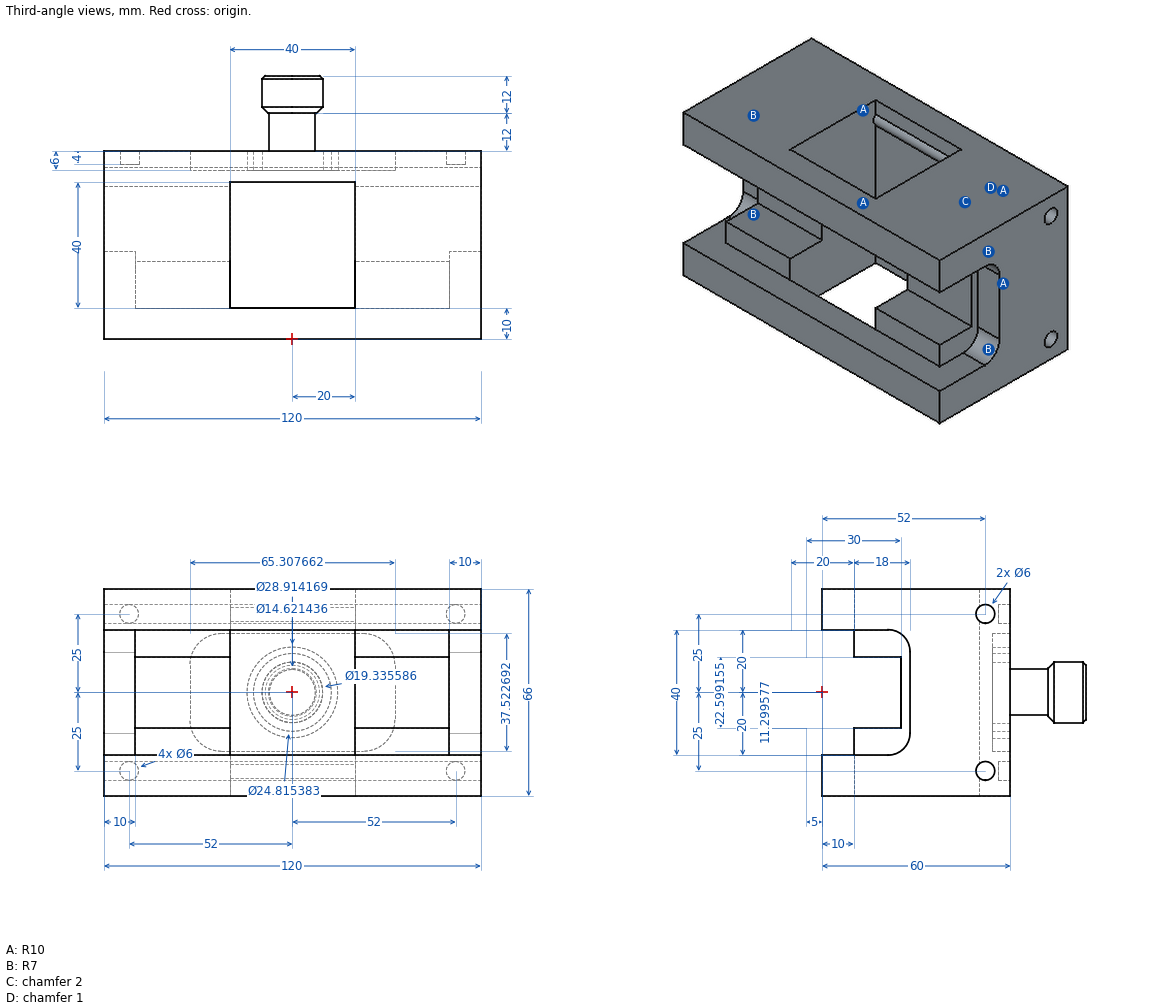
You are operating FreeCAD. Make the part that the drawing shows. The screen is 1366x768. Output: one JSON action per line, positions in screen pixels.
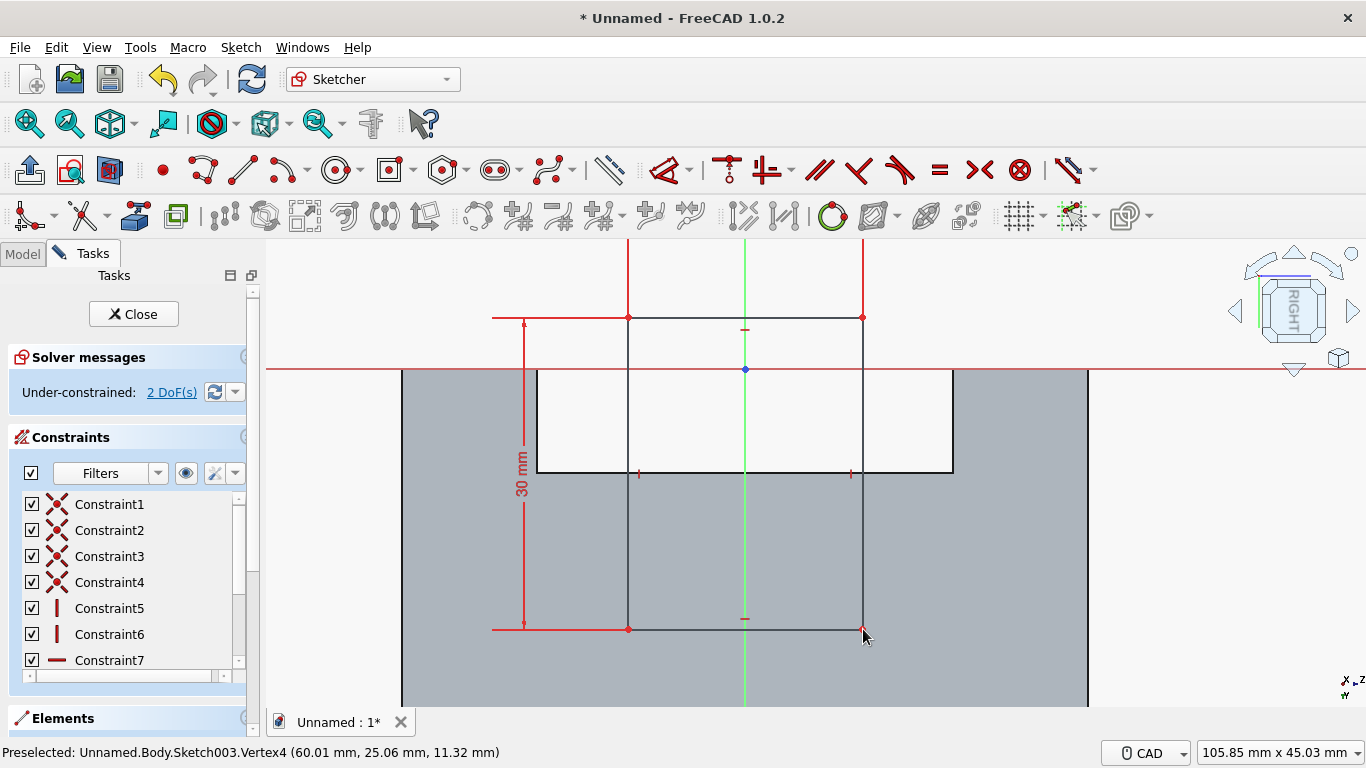
{"action": "left_click", "coordinate": [664, 170]}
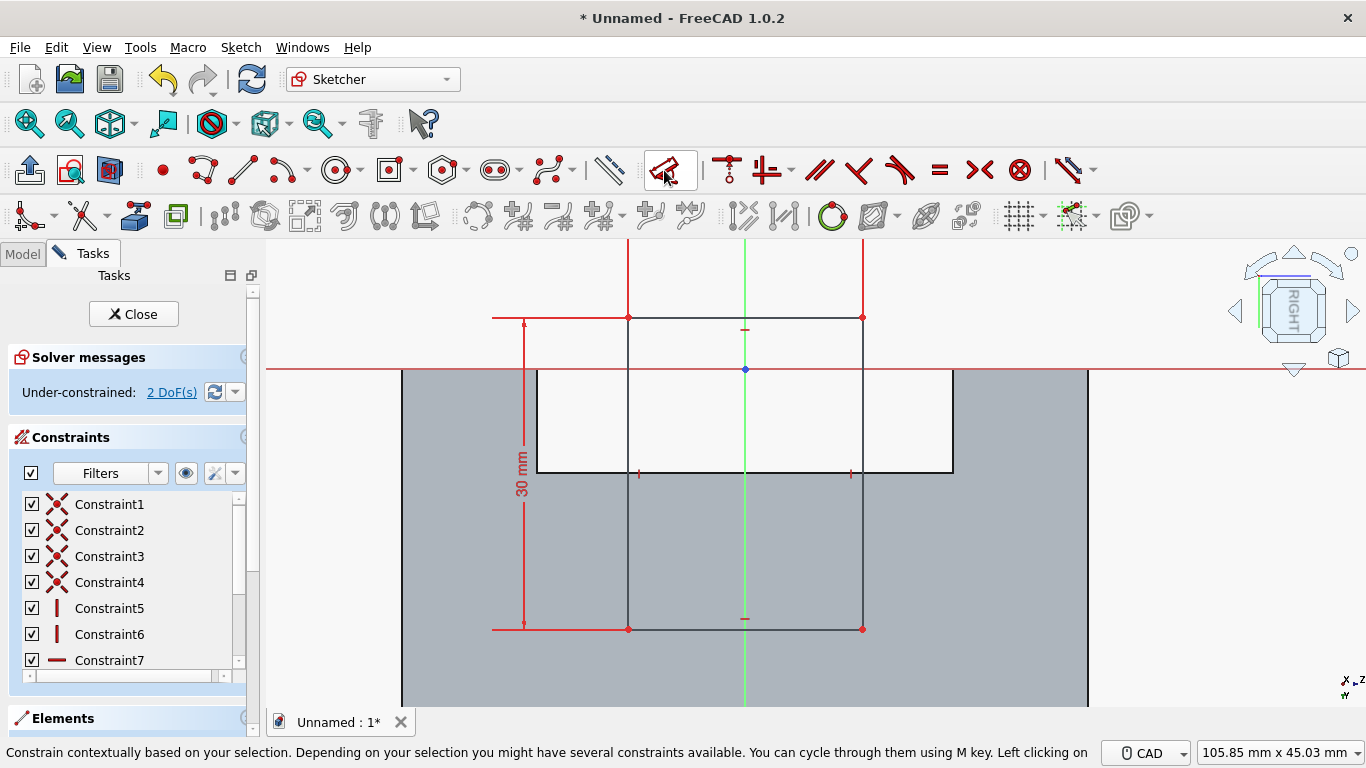
{"action": "left_click", "coordinate": [628, 318]}
{"action": "left_click", "coordinate": [594, 344]}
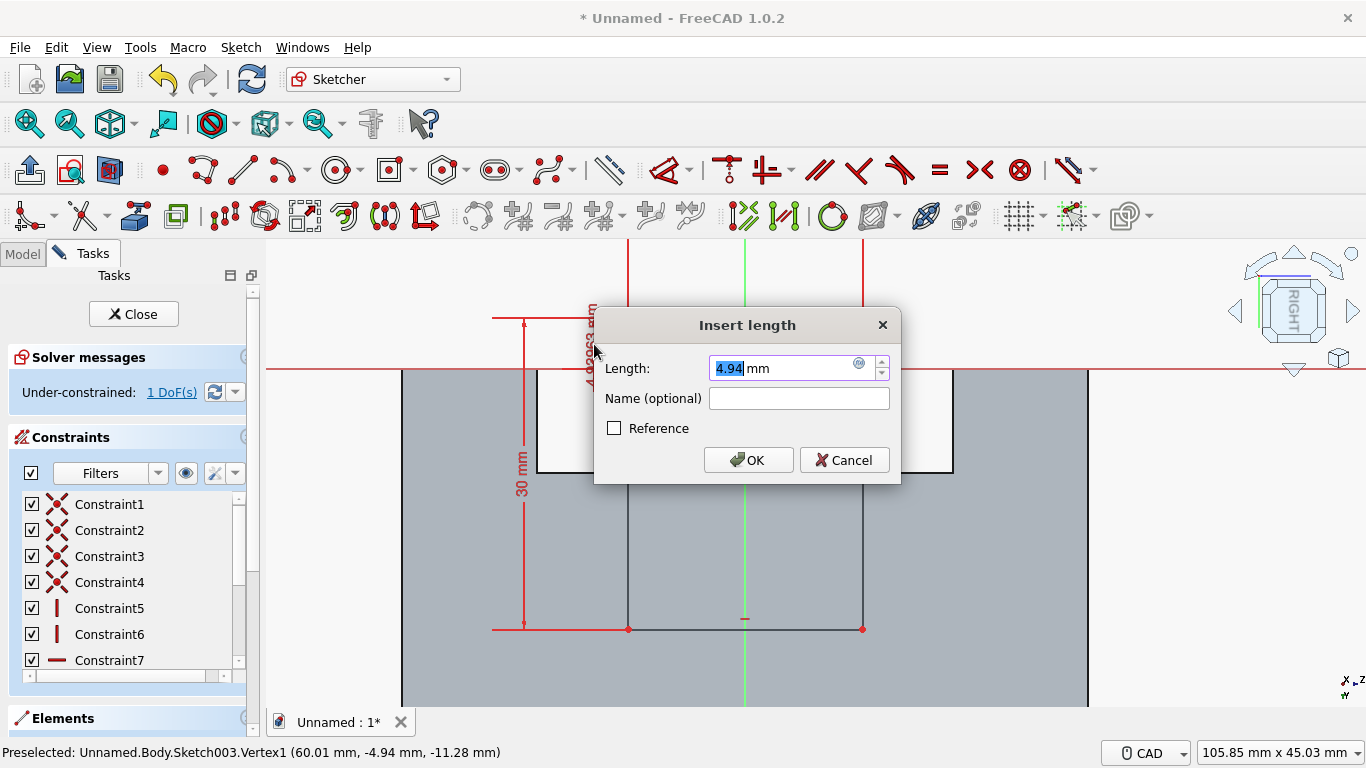
{"action": "type", "text": "5"}
{"action": "key", "text": "Return"}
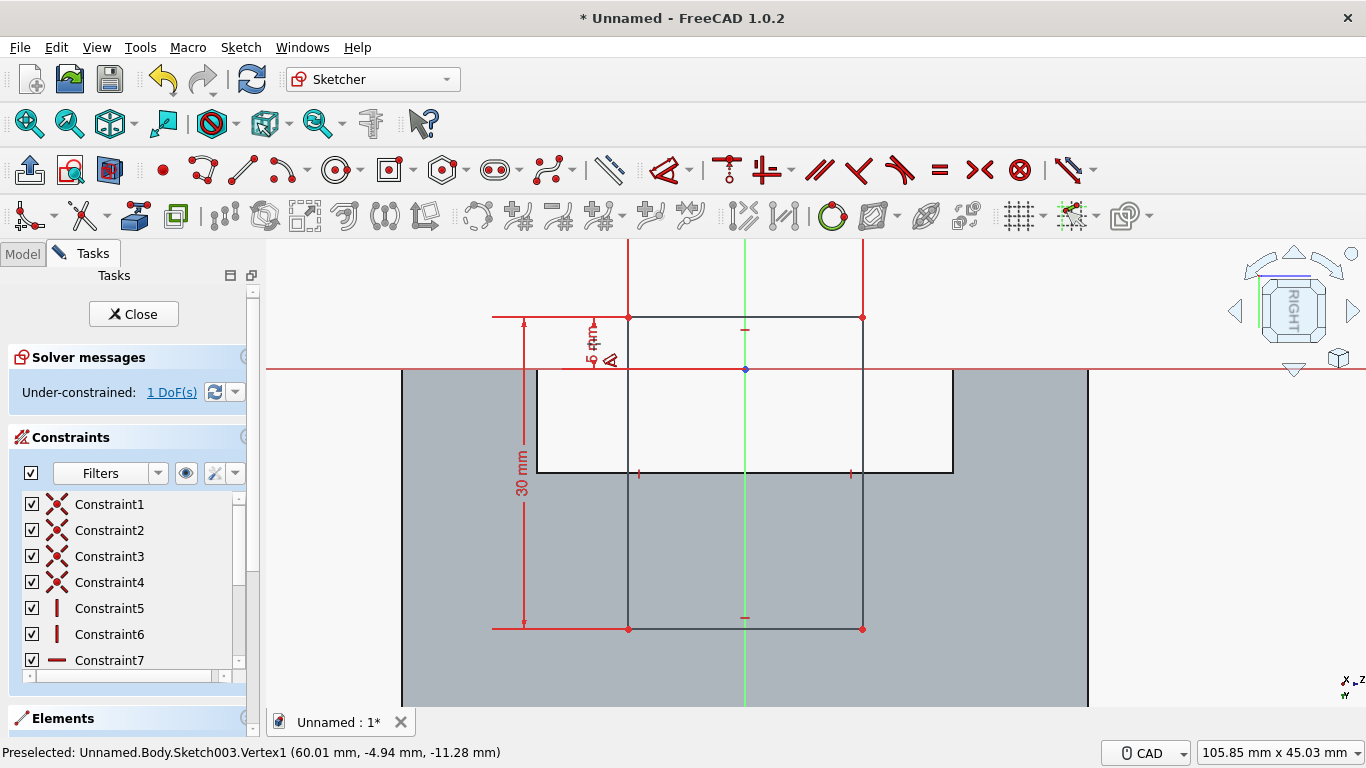
{"action": "left_click", "coordinate": [628, 317]}
{"action": "left_click", "coordinate": [687, 283]}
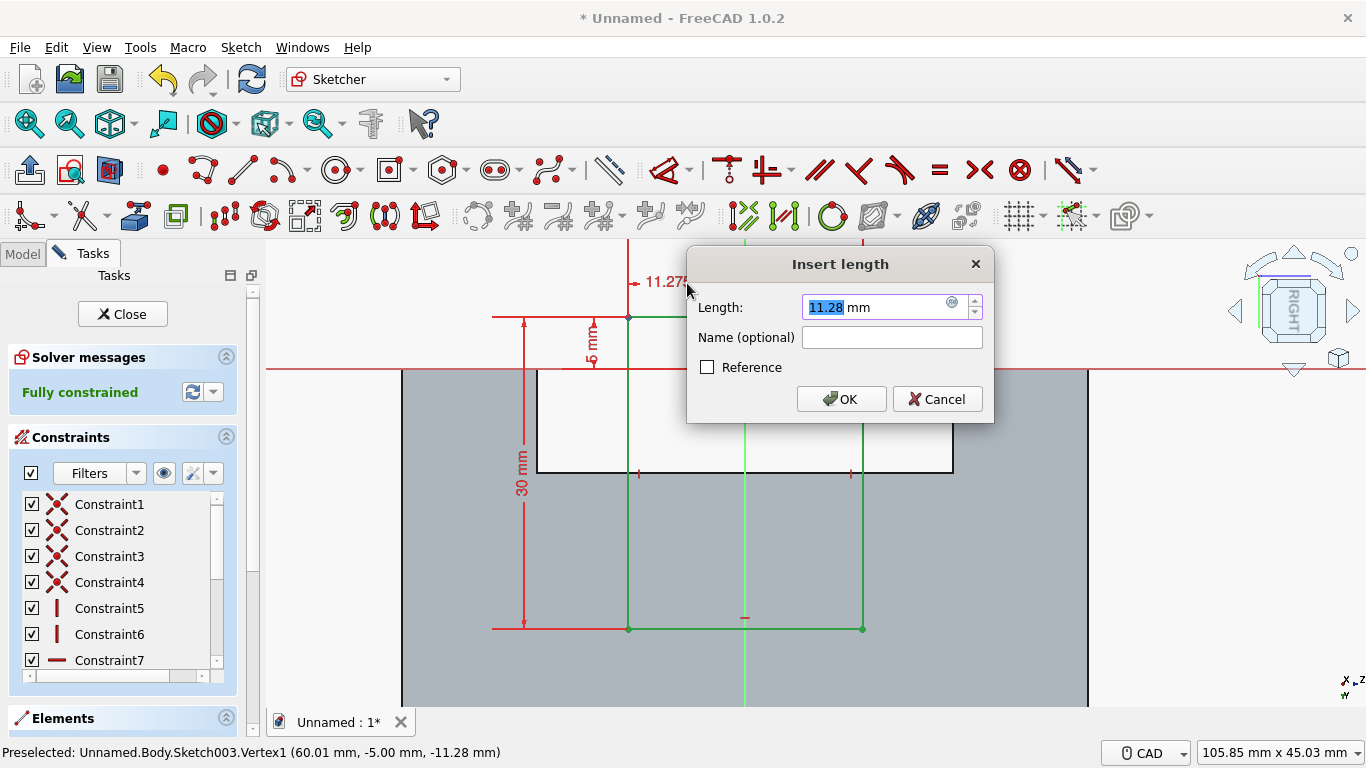
{"action": "type", "text": "11.299577"}
{"action": "key", "text": "Return"}
{"action": "key", "text": "Escape"}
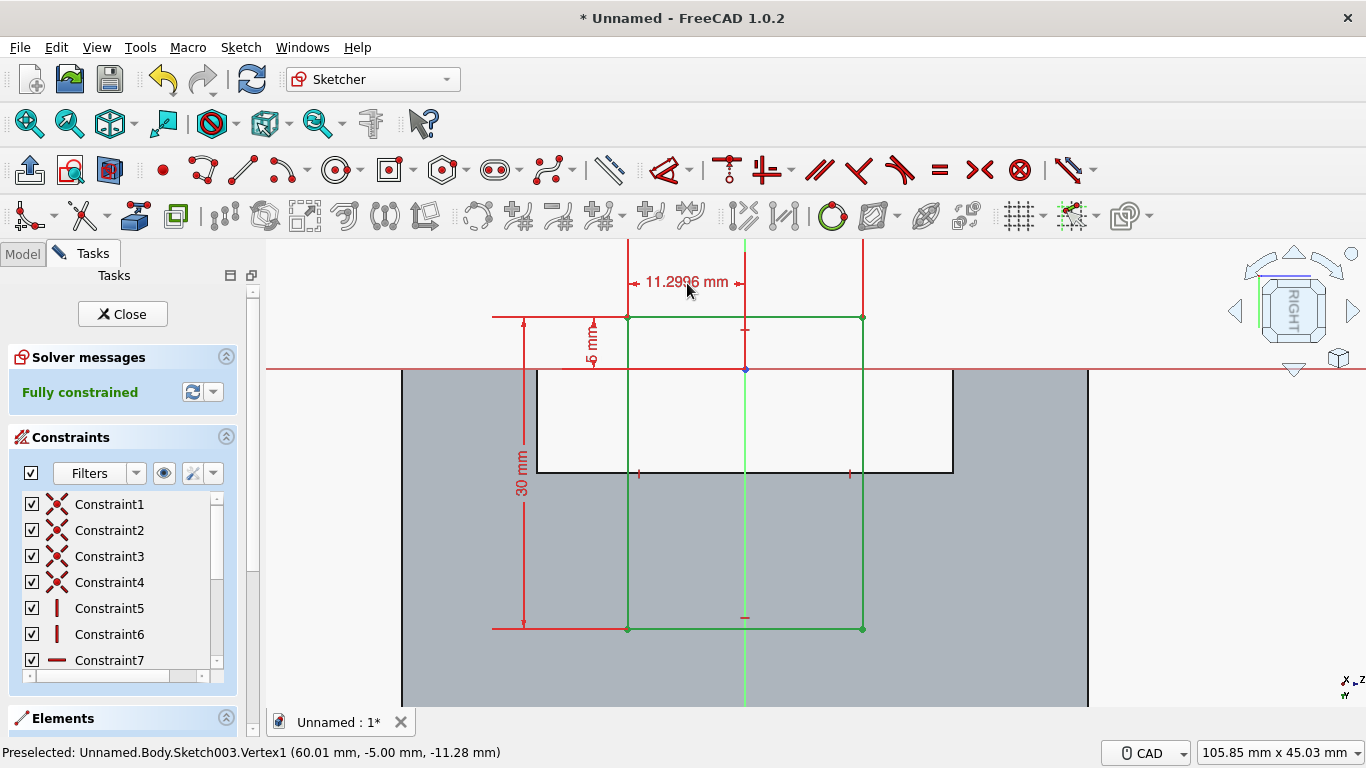
{"action": "left_click", "coordinate": [123, 314]}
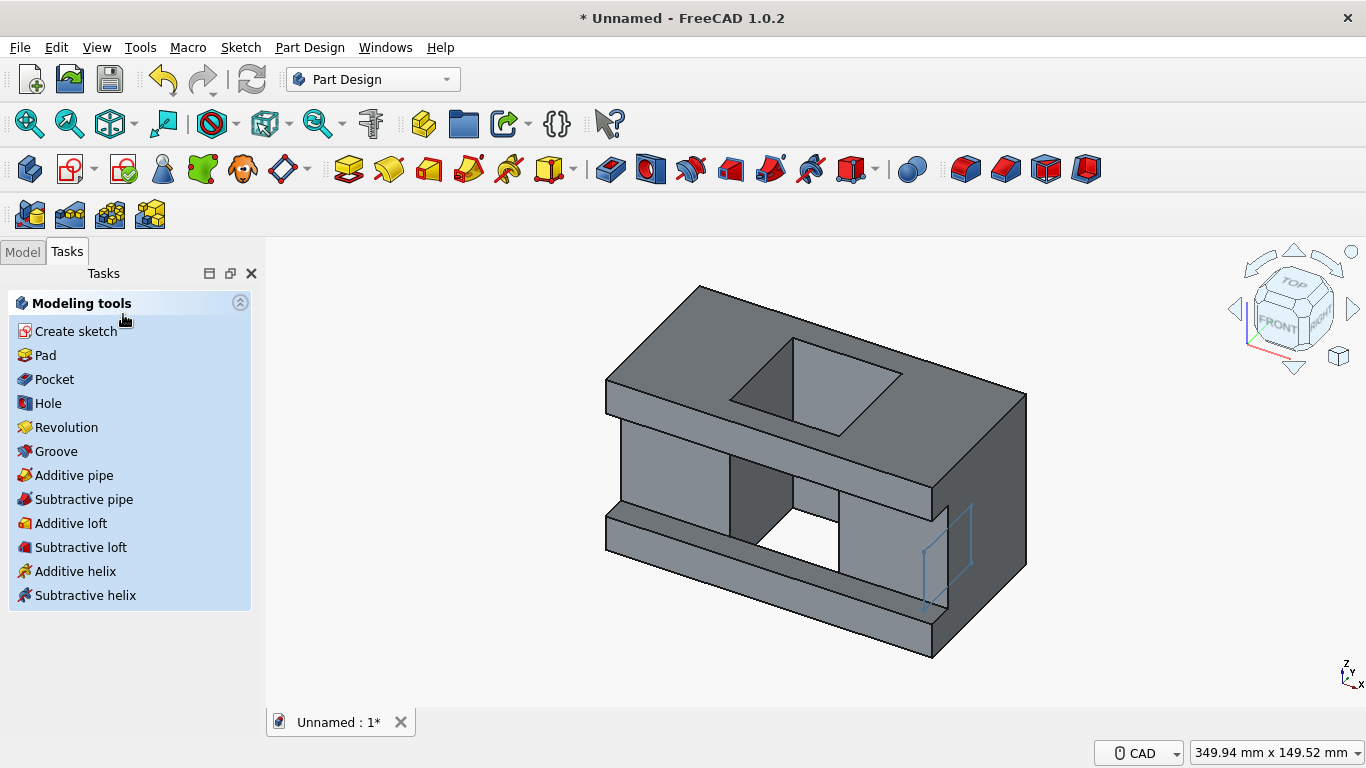
{"action": "left_click", "coordinate": [612, 170]}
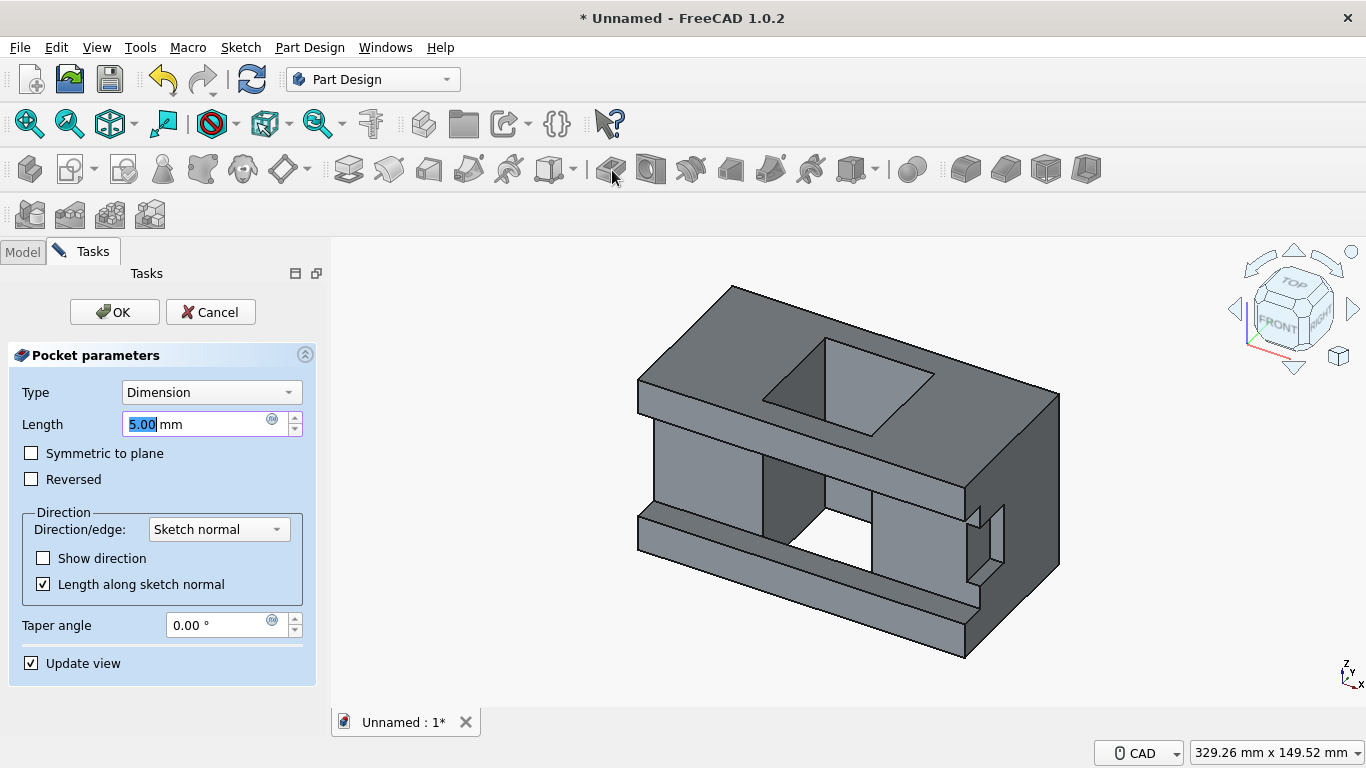
{"action": "type", "text": "120"}
{"action": "key", "text": "Tab"}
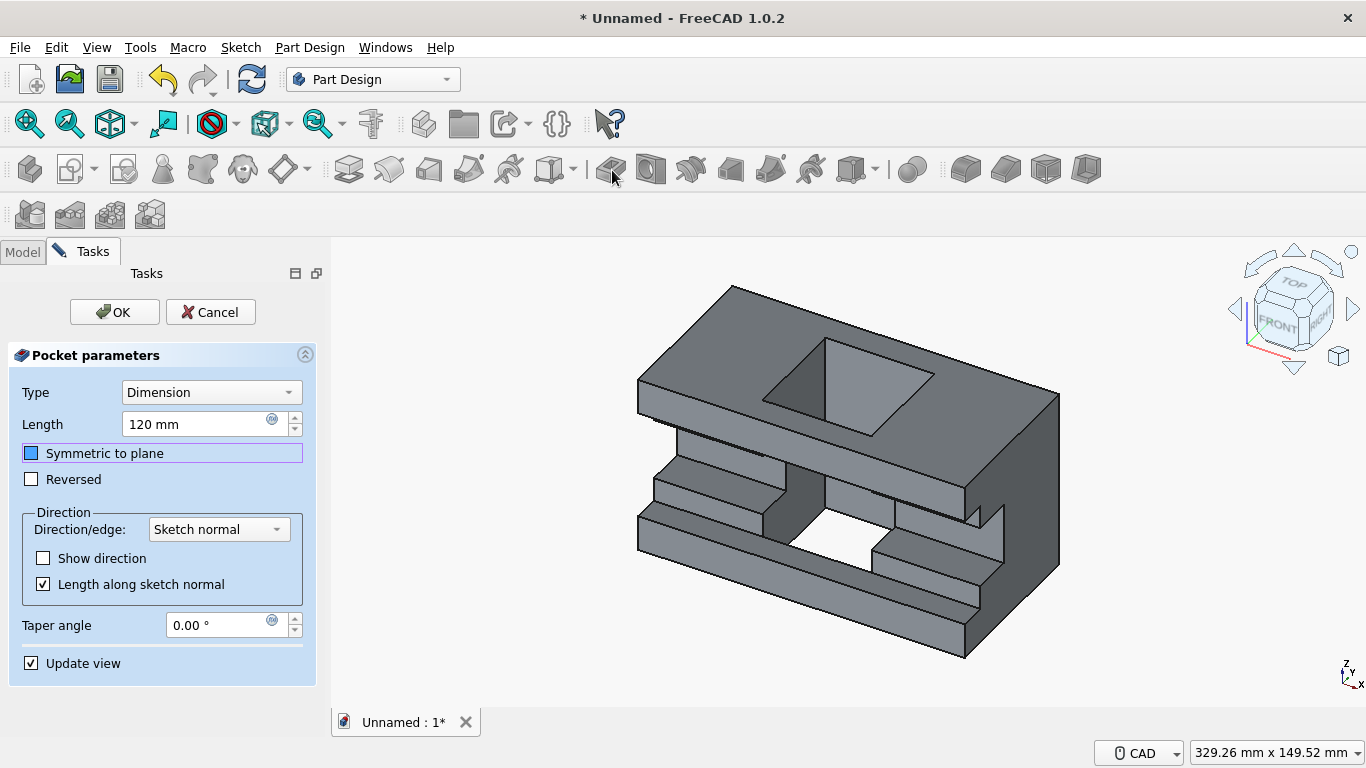
{"action": "left_click", "coordinate": [115, 312]}